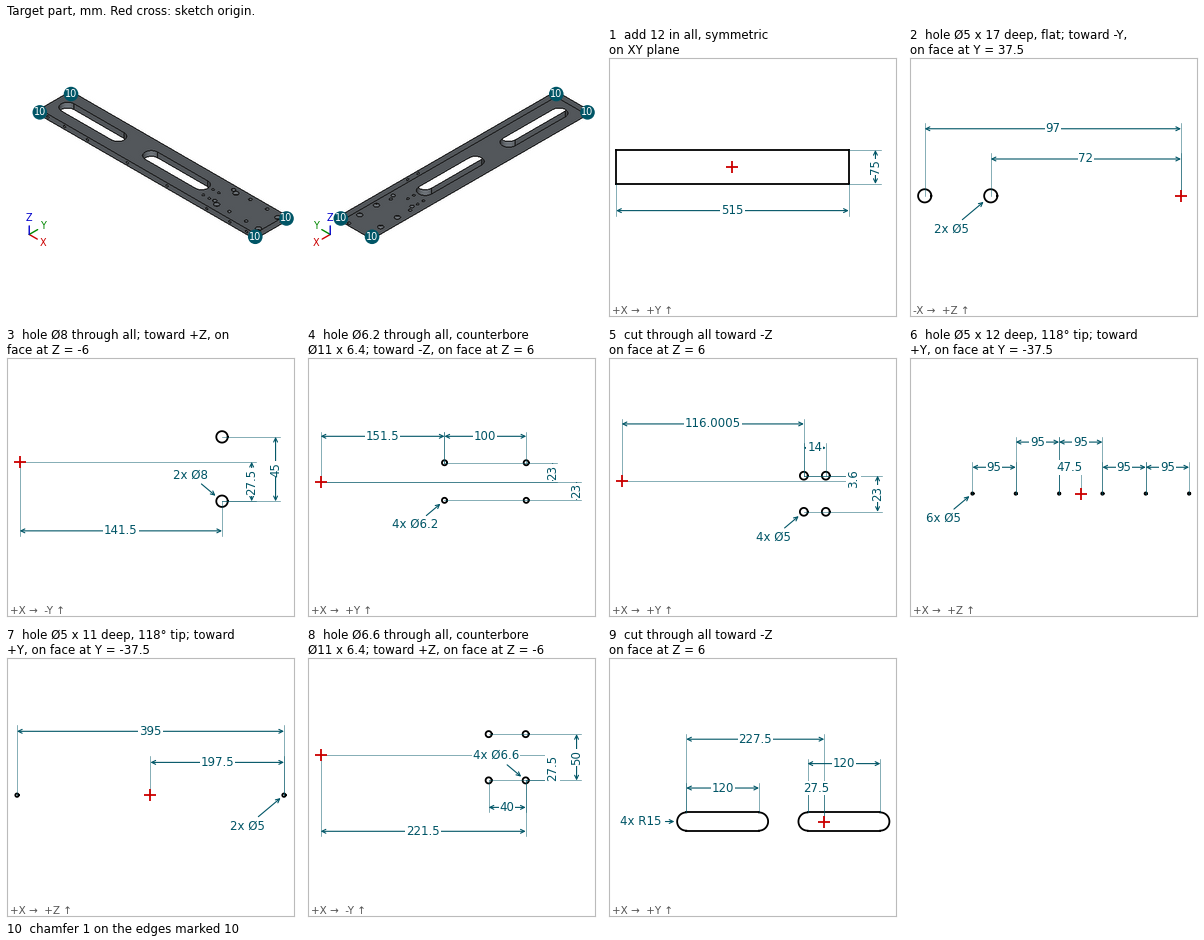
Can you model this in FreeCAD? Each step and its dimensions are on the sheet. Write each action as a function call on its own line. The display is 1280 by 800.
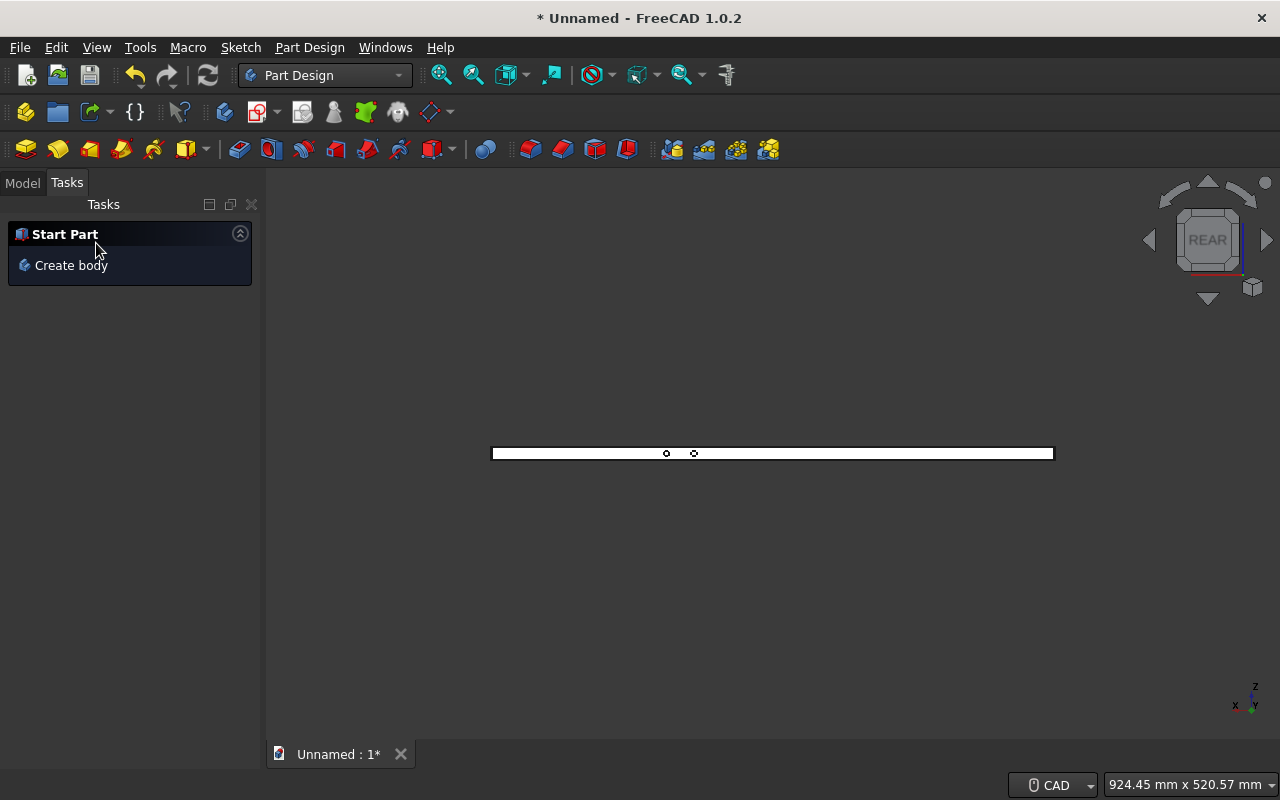
key(0)